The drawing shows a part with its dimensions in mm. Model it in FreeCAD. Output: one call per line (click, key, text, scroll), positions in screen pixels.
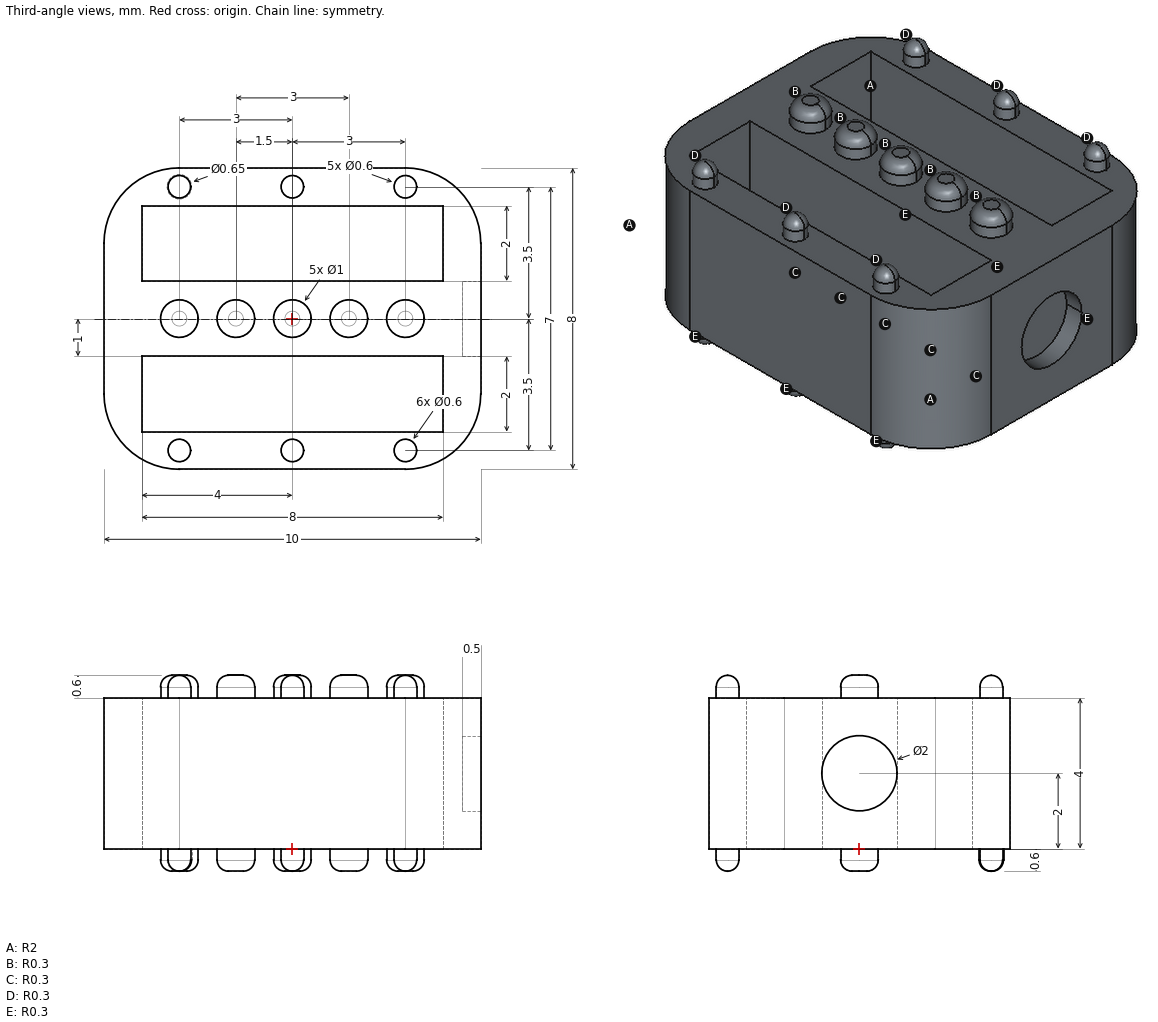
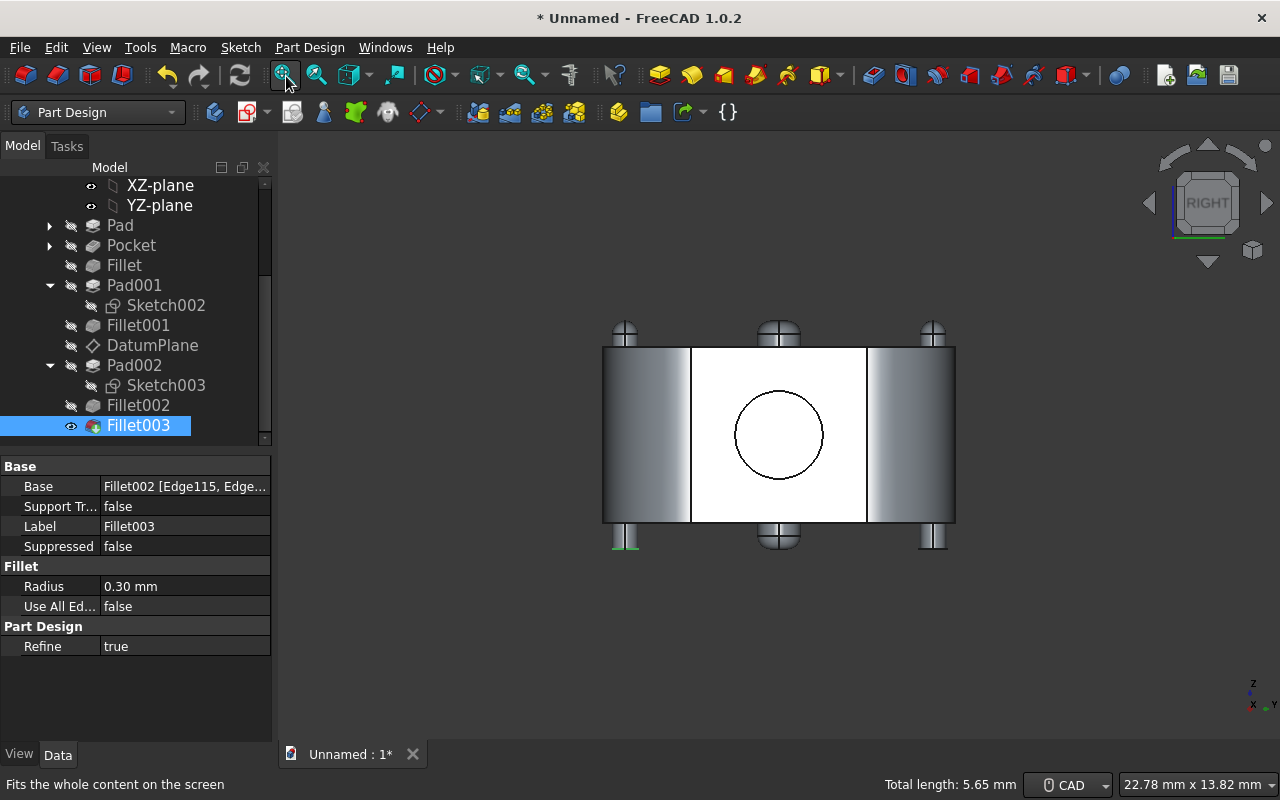
click(941, 548, ctrl)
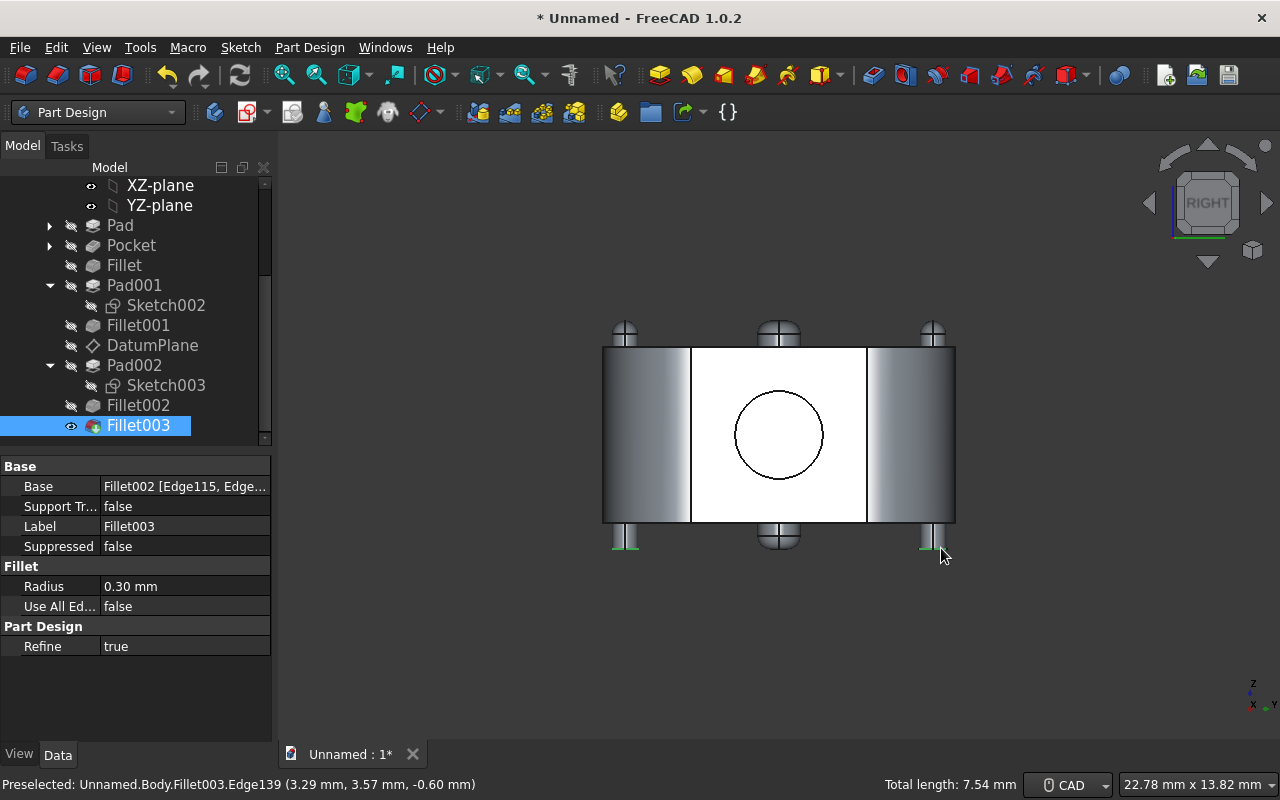
key(5)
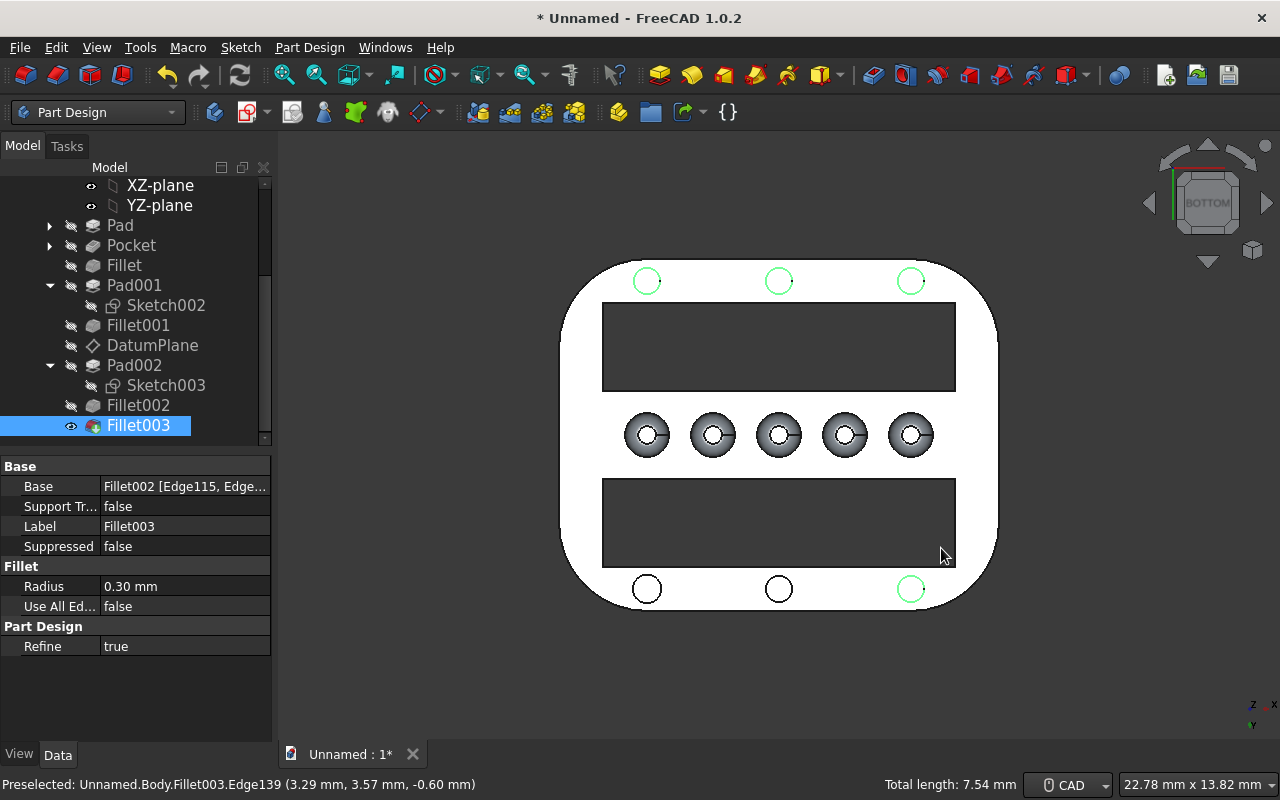
click(766, 588, ctrl)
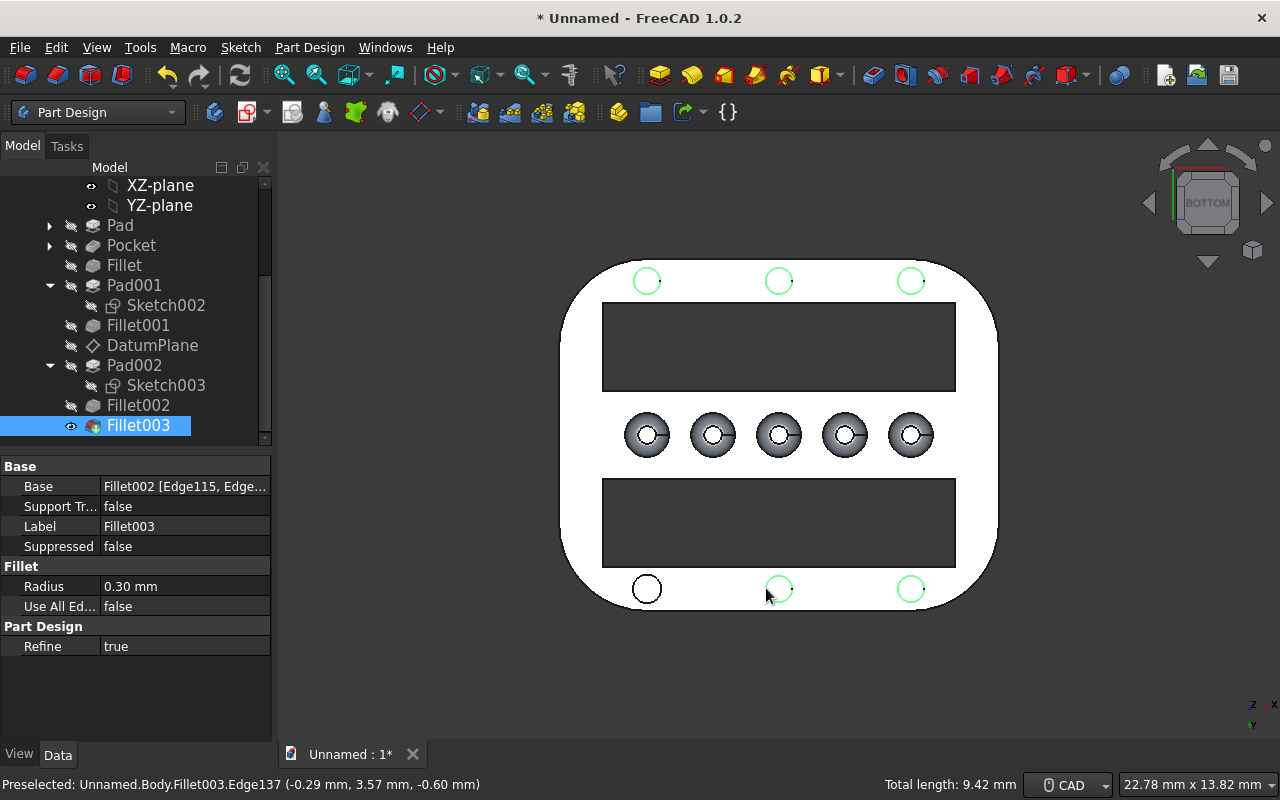
click(633, 588, ctrl)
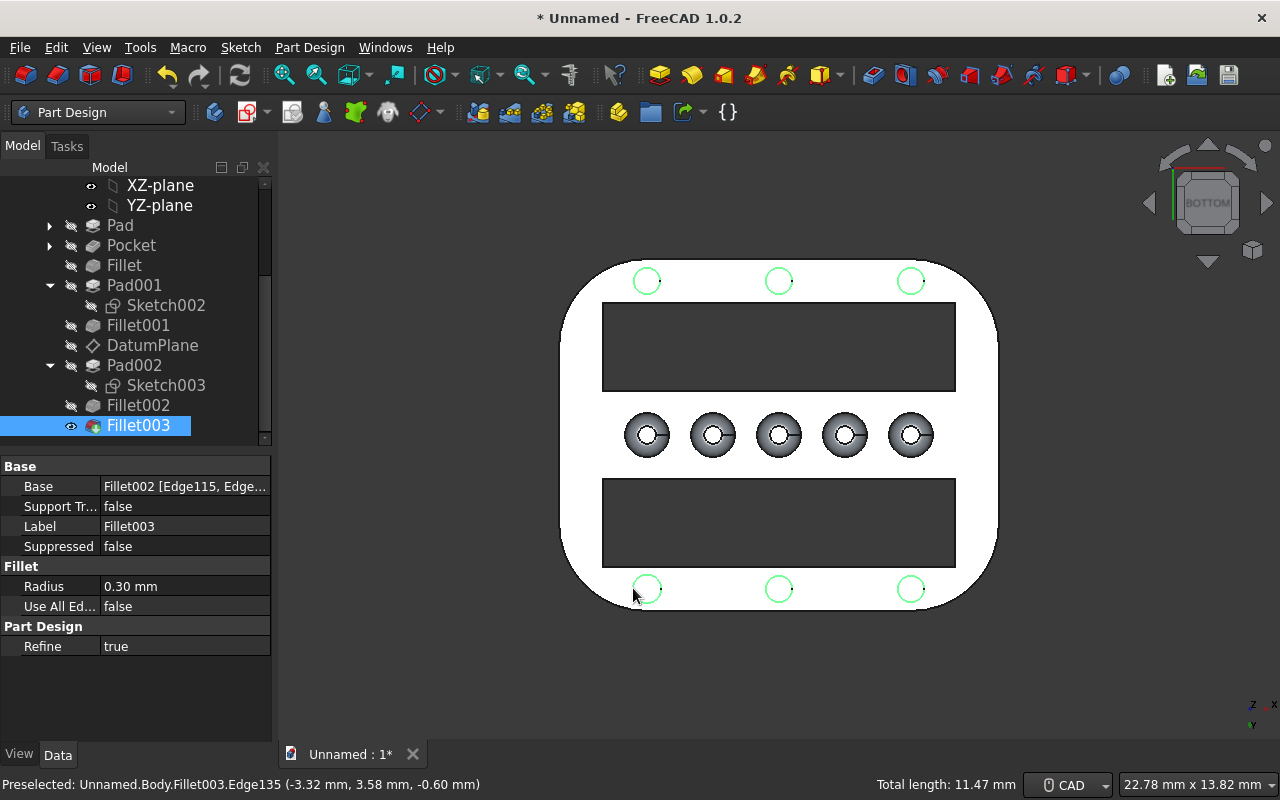
click(26, 76)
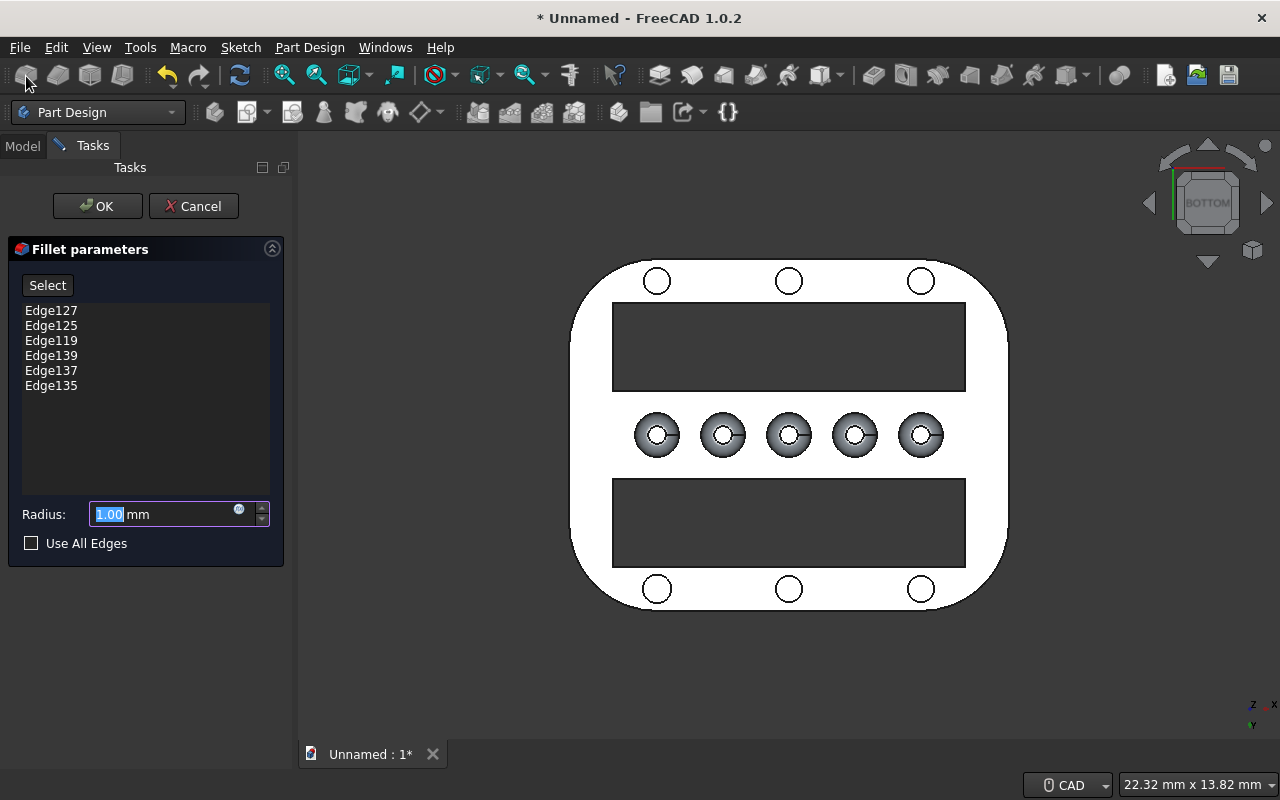
text(0.3)
key(Tab)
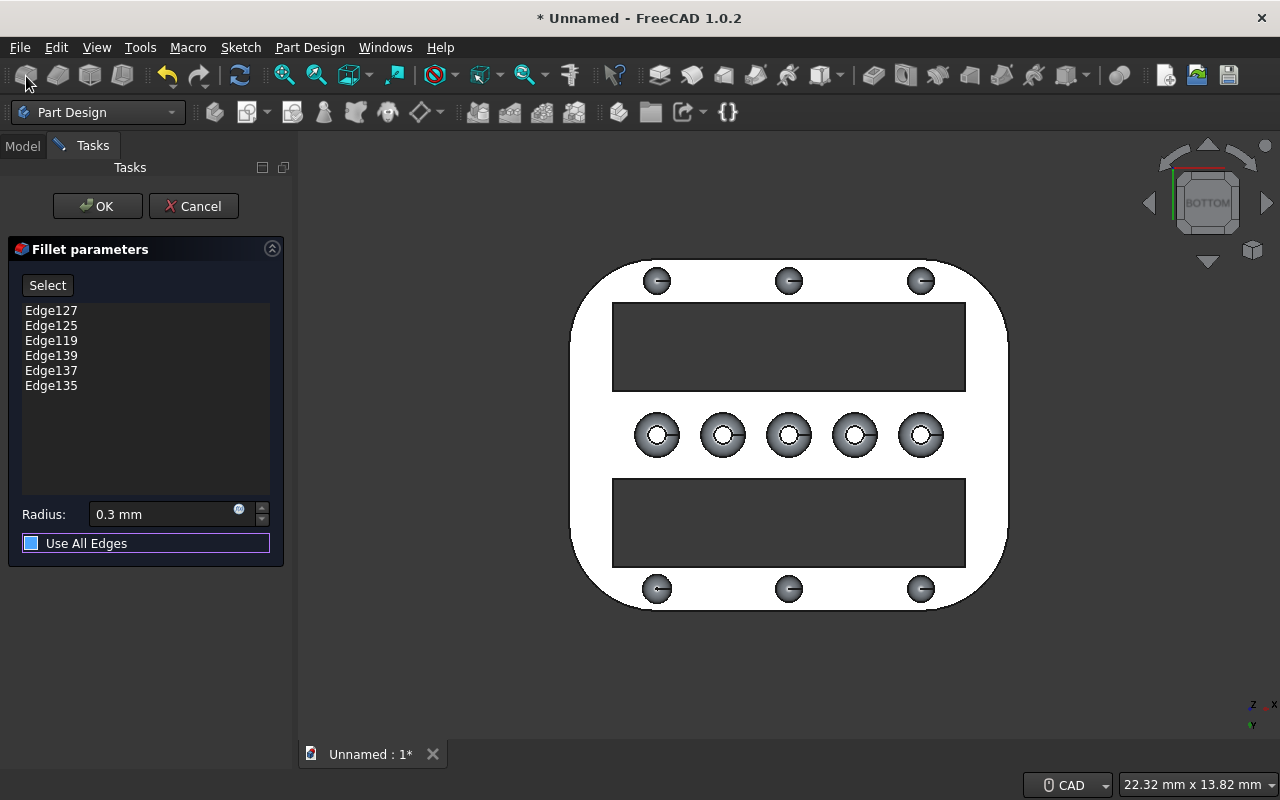
click(98, 206)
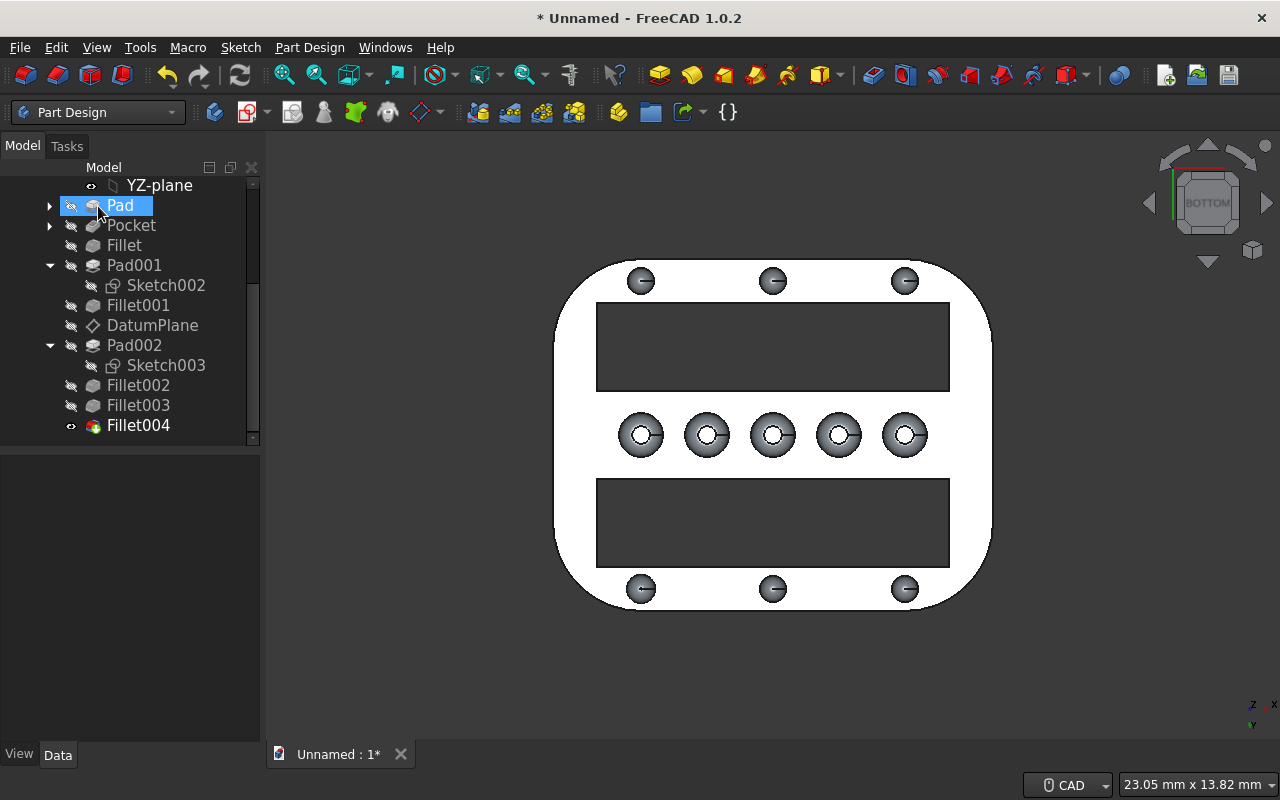
key(0)